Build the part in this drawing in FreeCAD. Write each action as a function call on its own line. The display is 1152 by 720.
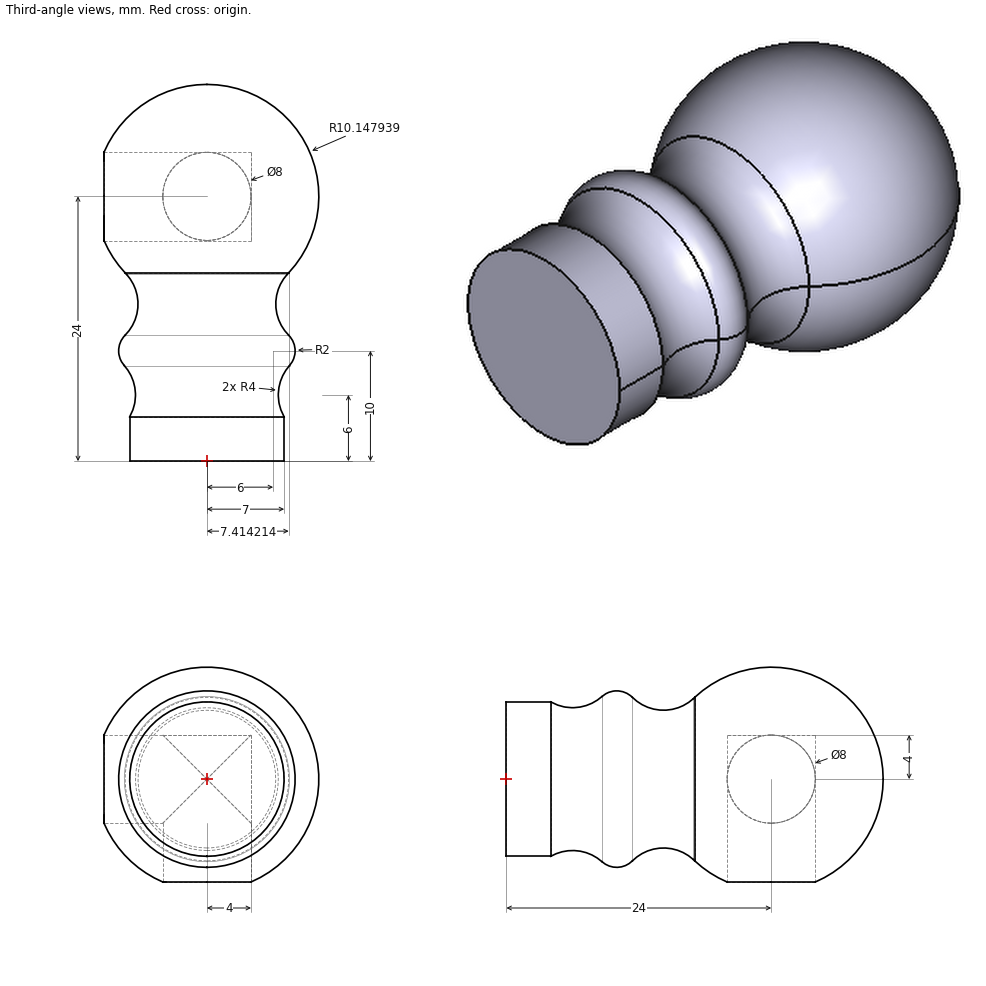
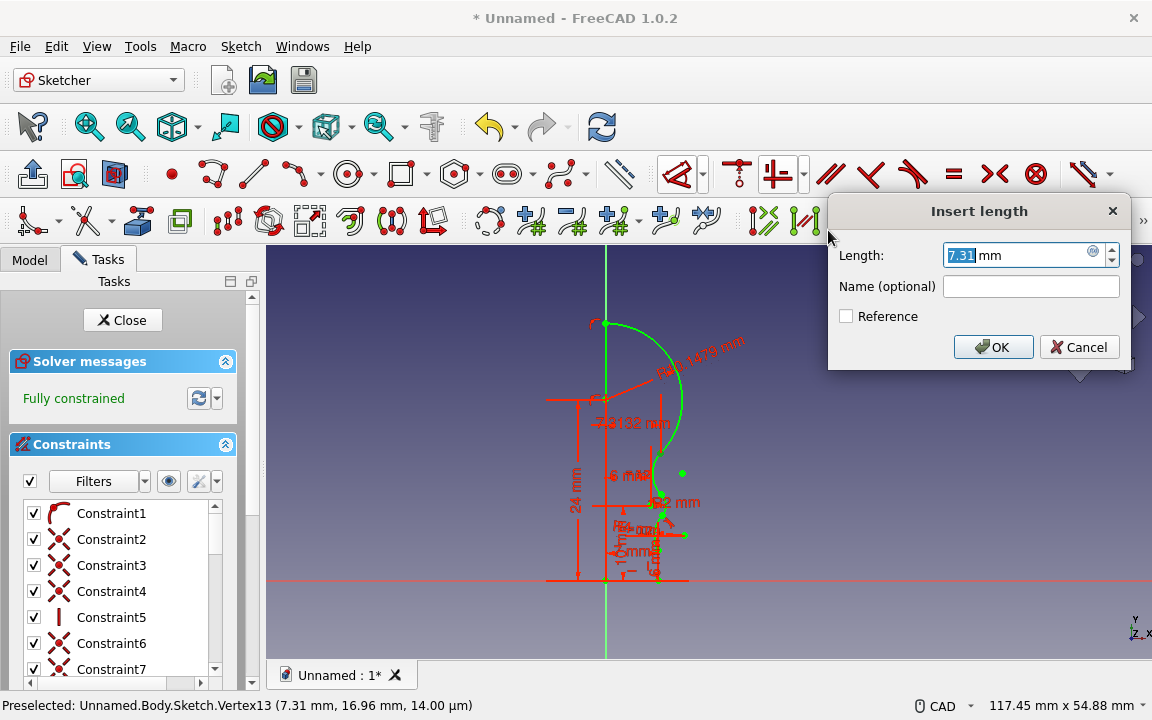
text(7.414214)
key(Return)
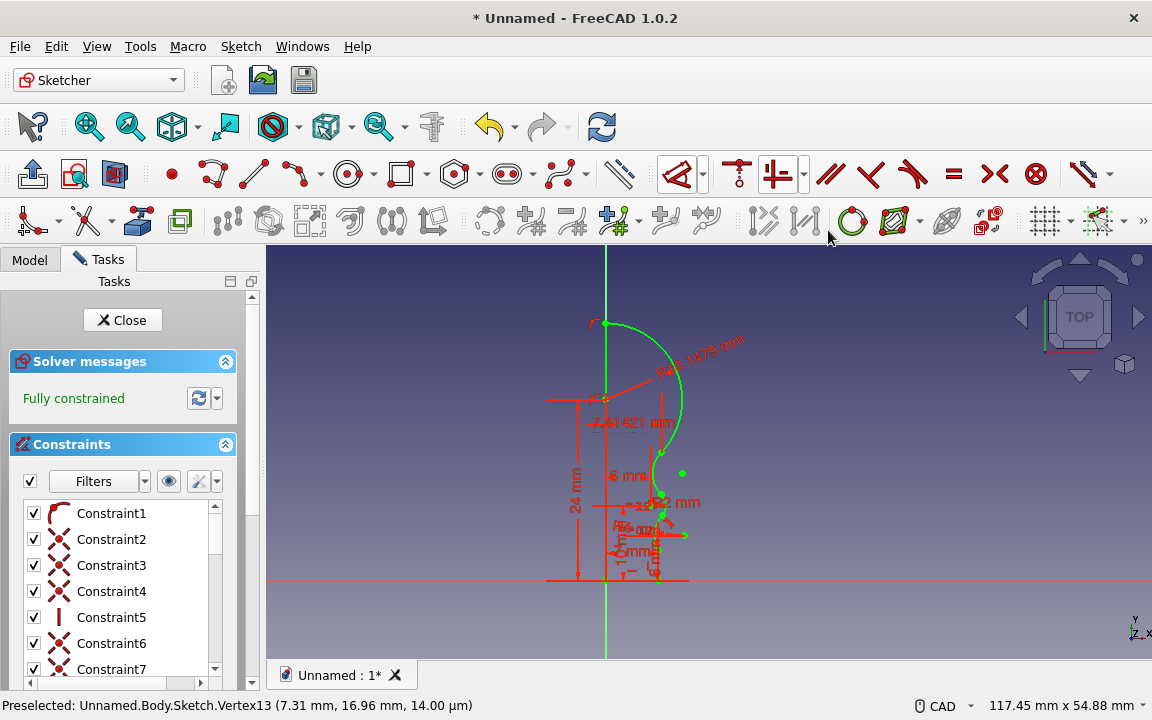
click(123, 320)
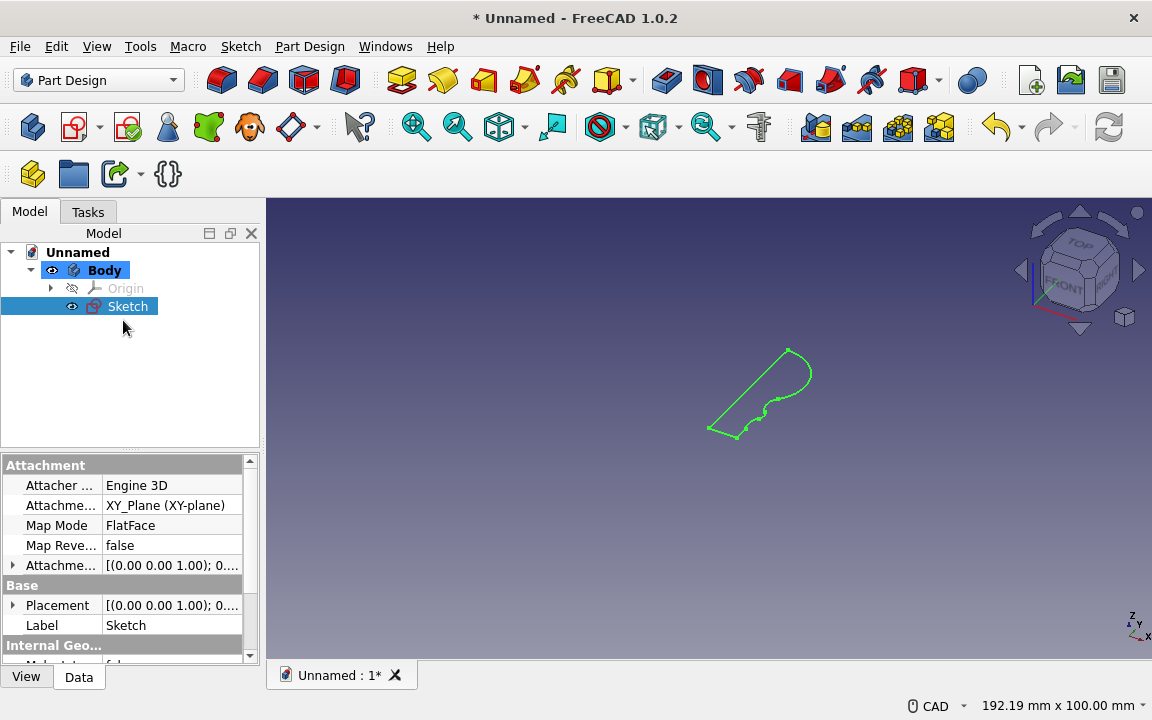
click(443, 80)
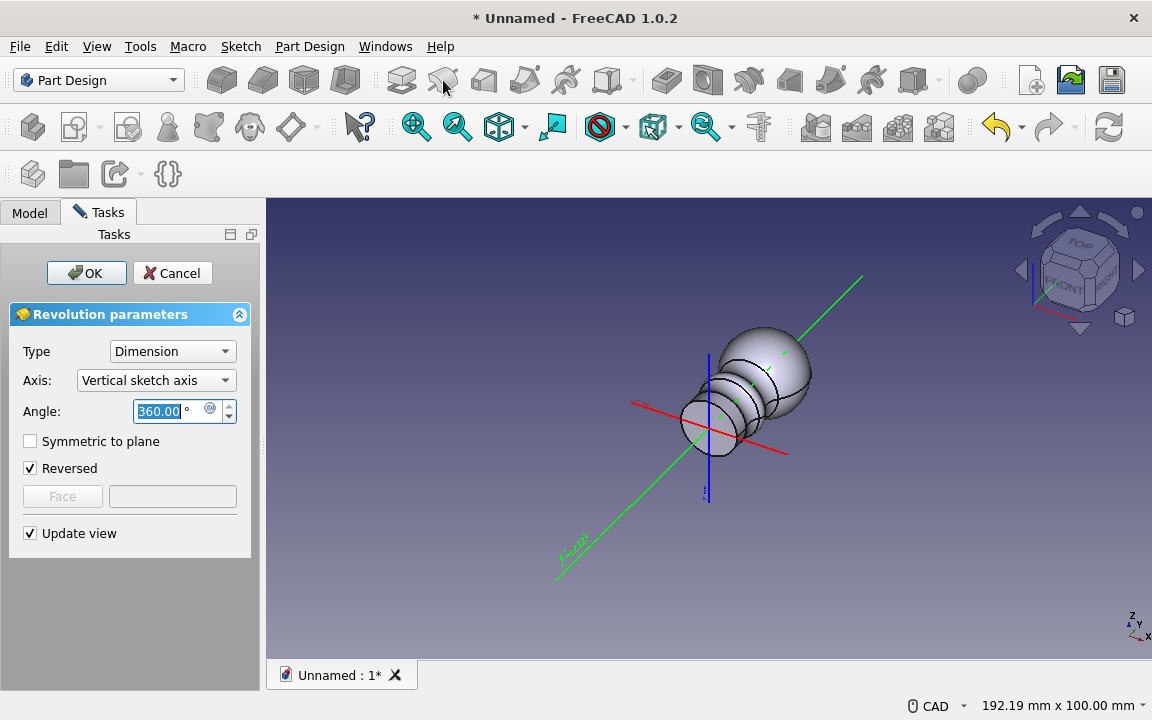
click(87, 273)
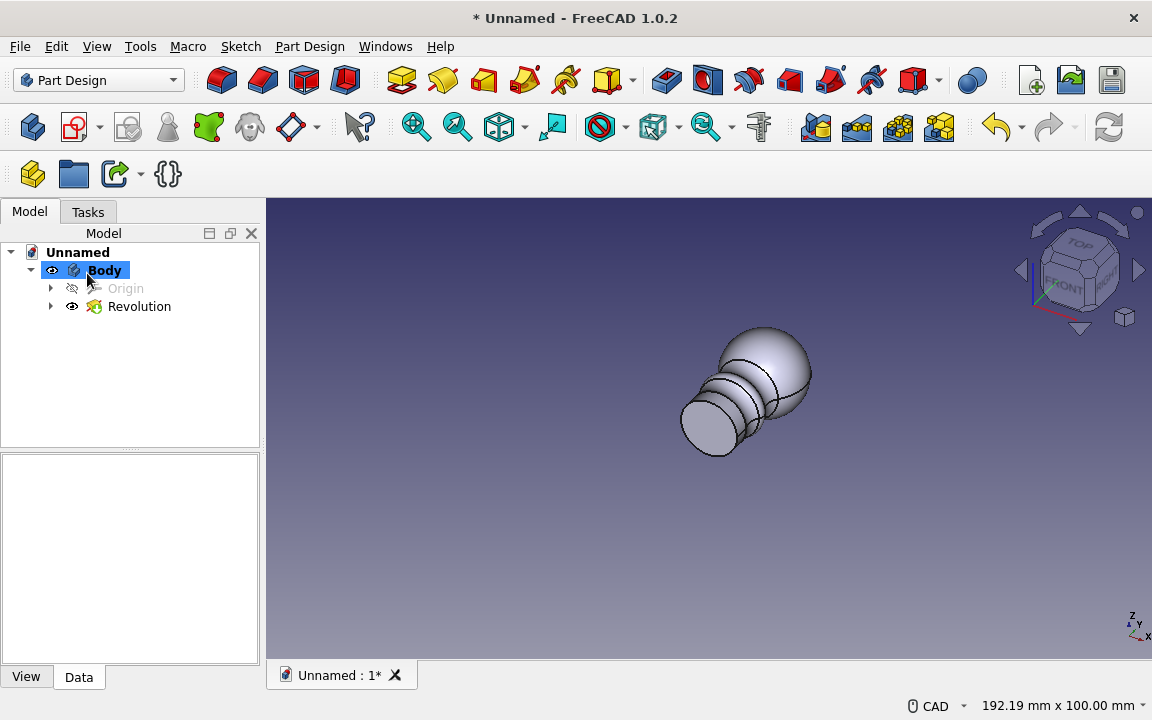
click(417, 128)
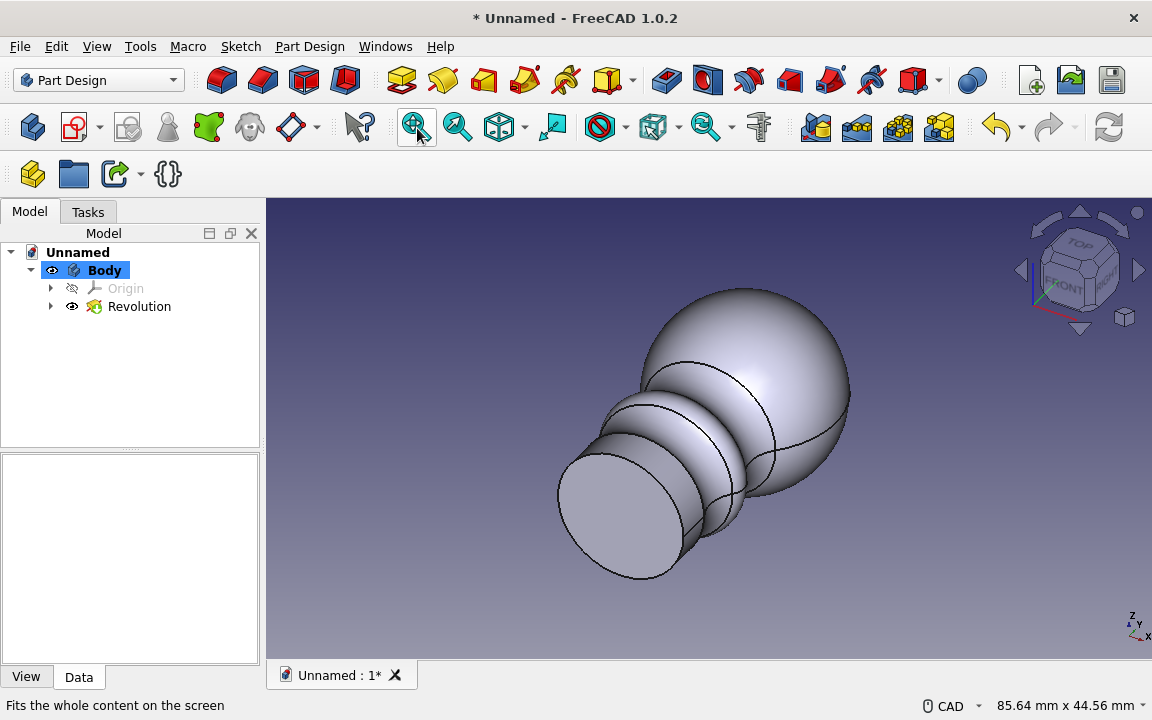
click(74, 128)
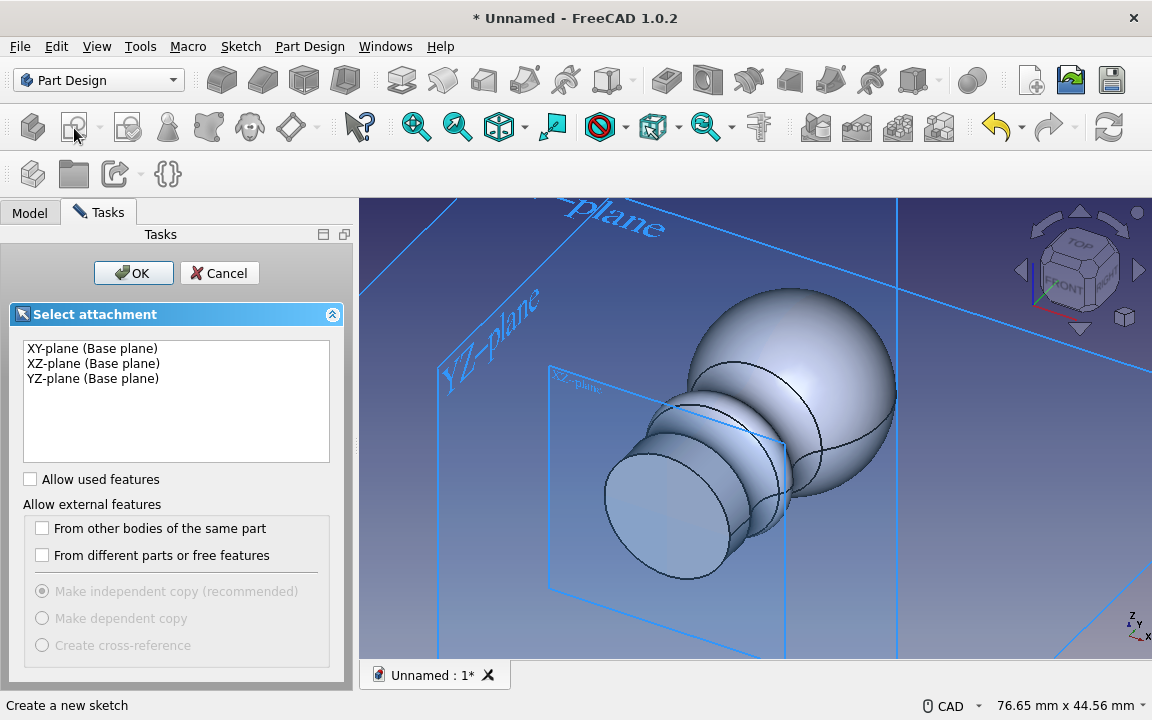
click(84, 348)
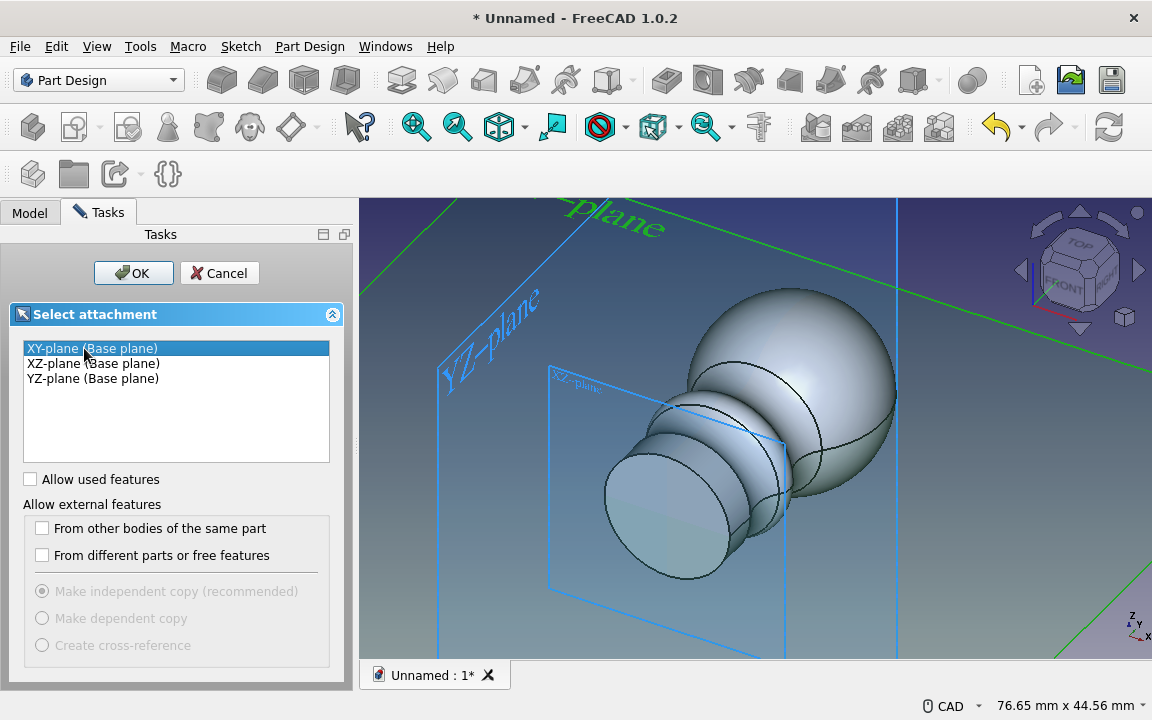
click(134, 273)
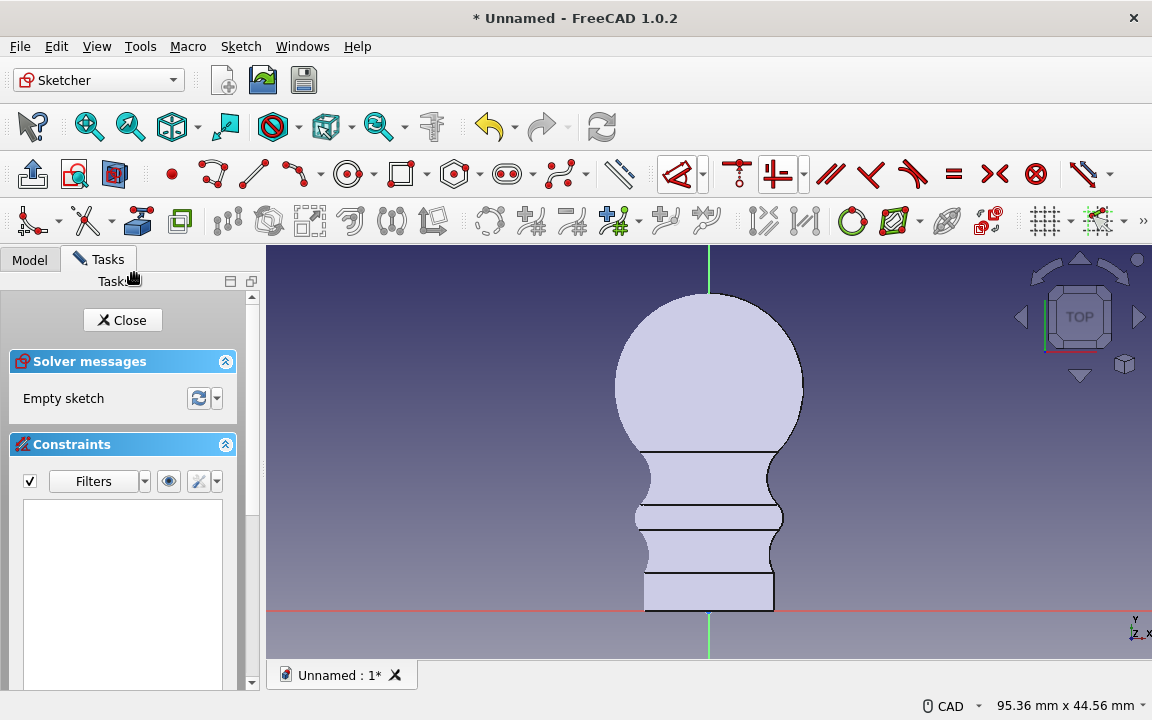
click(115, 174)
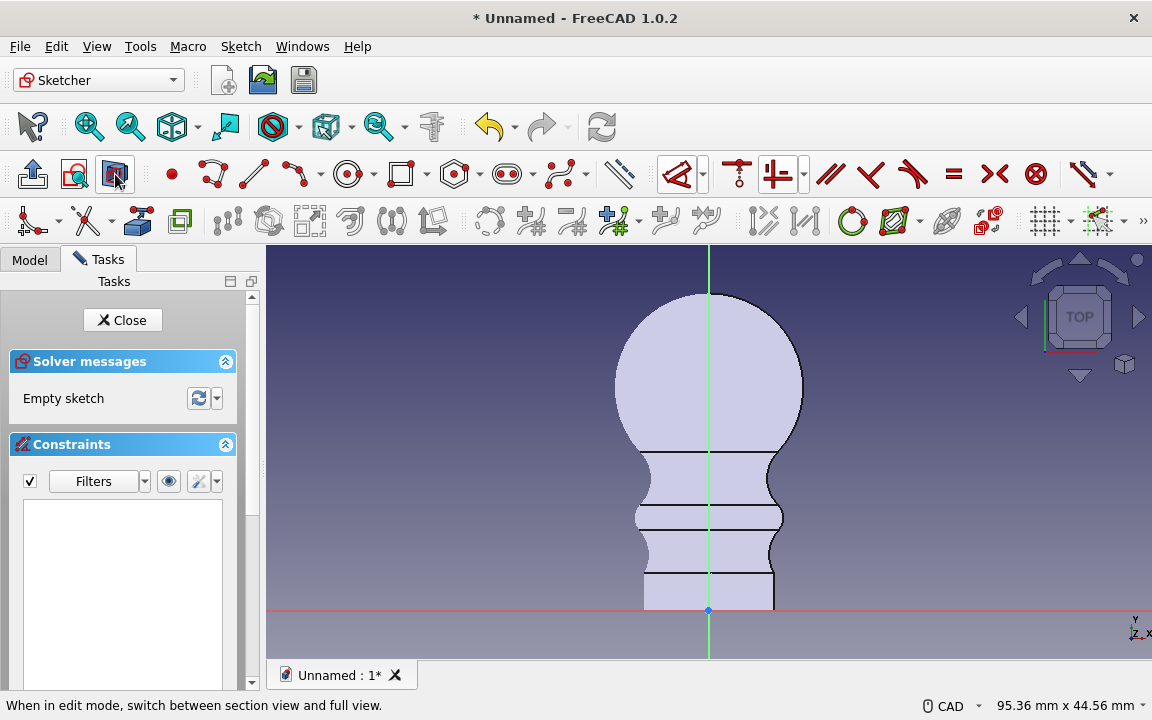
scroll(739, 360, up, 6)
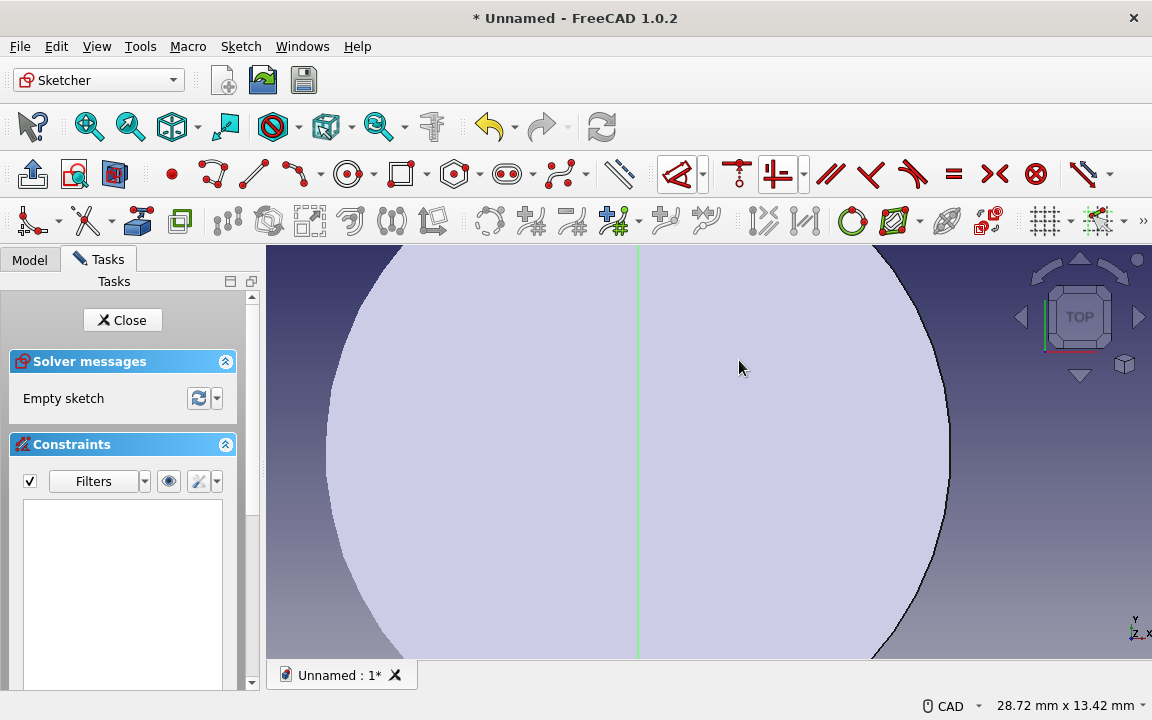
key(g)
key(c)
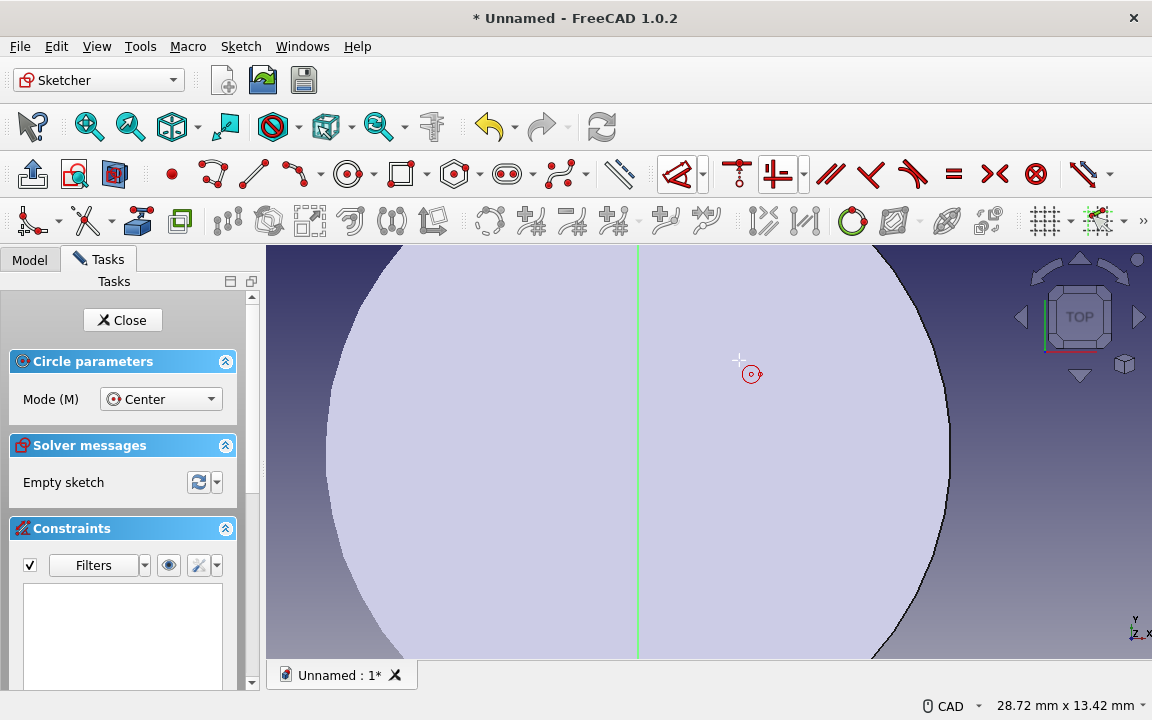
click(638, 451)
click(725, 364)
key(Escape)